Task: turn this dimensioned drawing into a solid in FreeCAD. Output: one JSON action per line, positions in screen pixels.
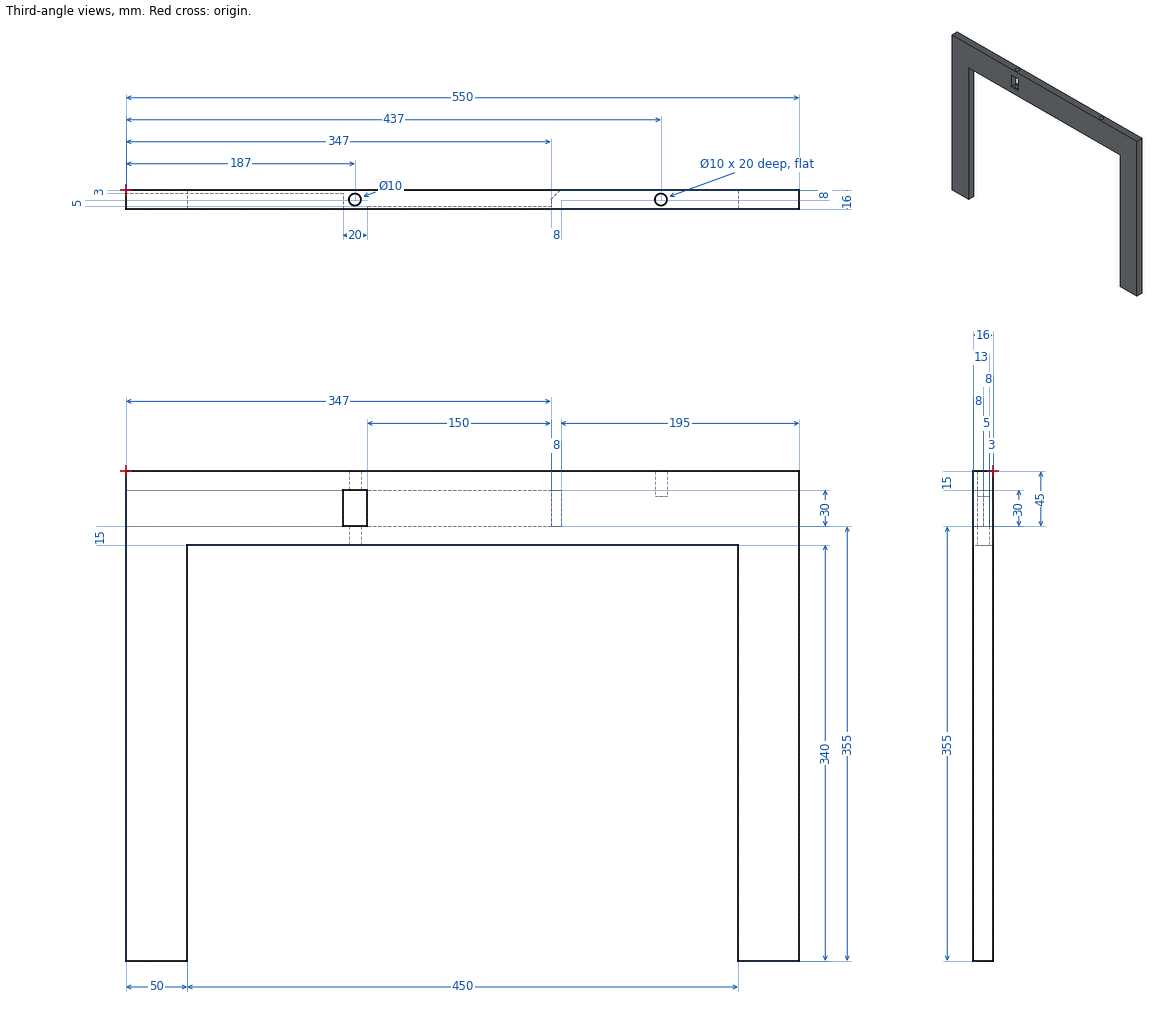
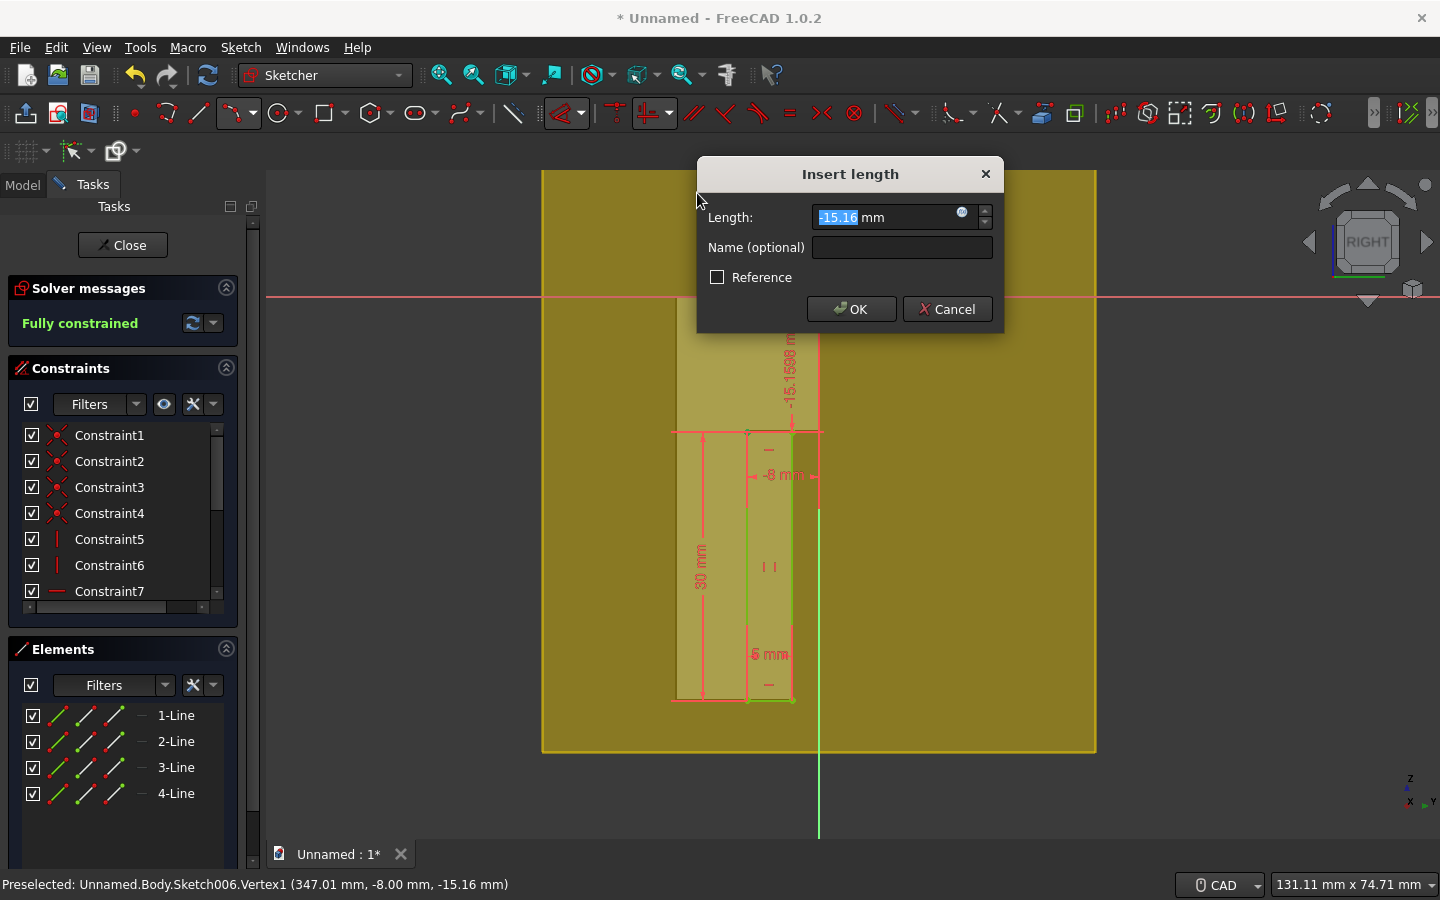
{"action": "type", "text": "-15"}
{"action": "key", "text": "Return"}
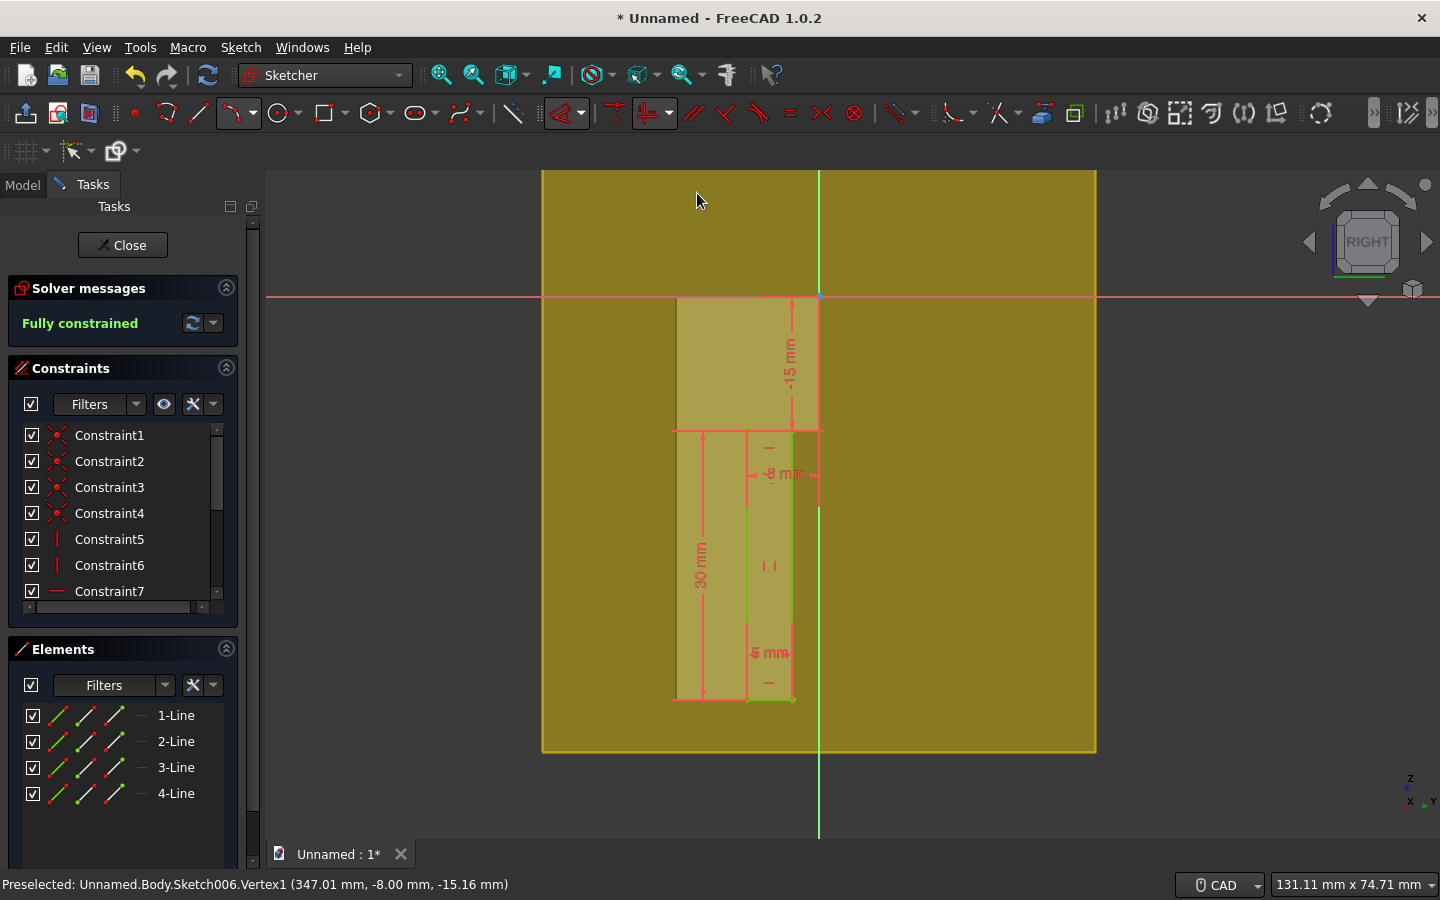
{"action": "left_click", "coordinate": [123, 245]}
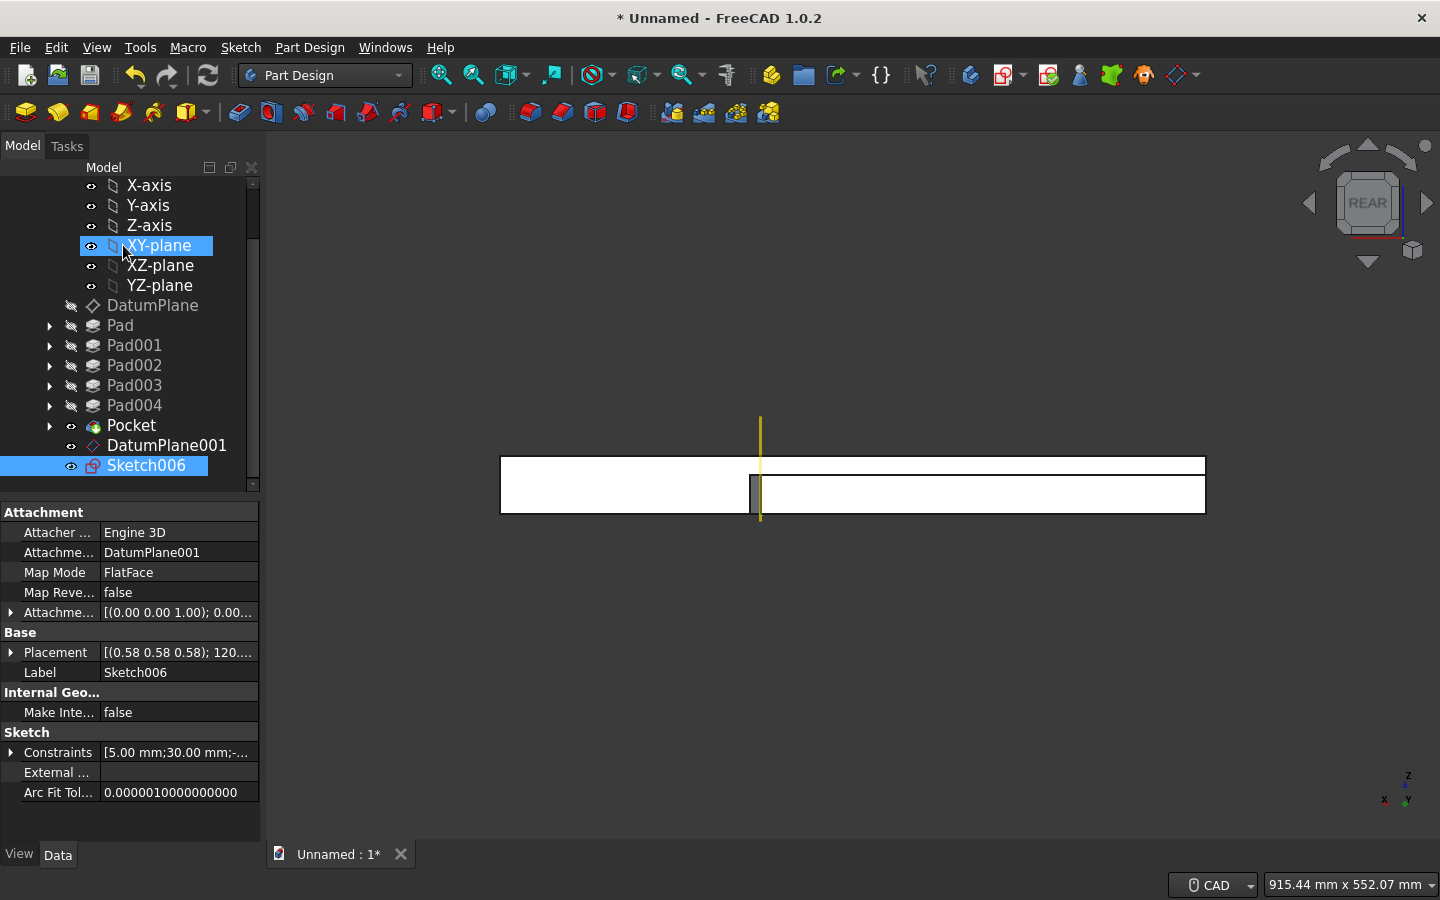
{"action": "left_click", "coordinate": [240, 112]}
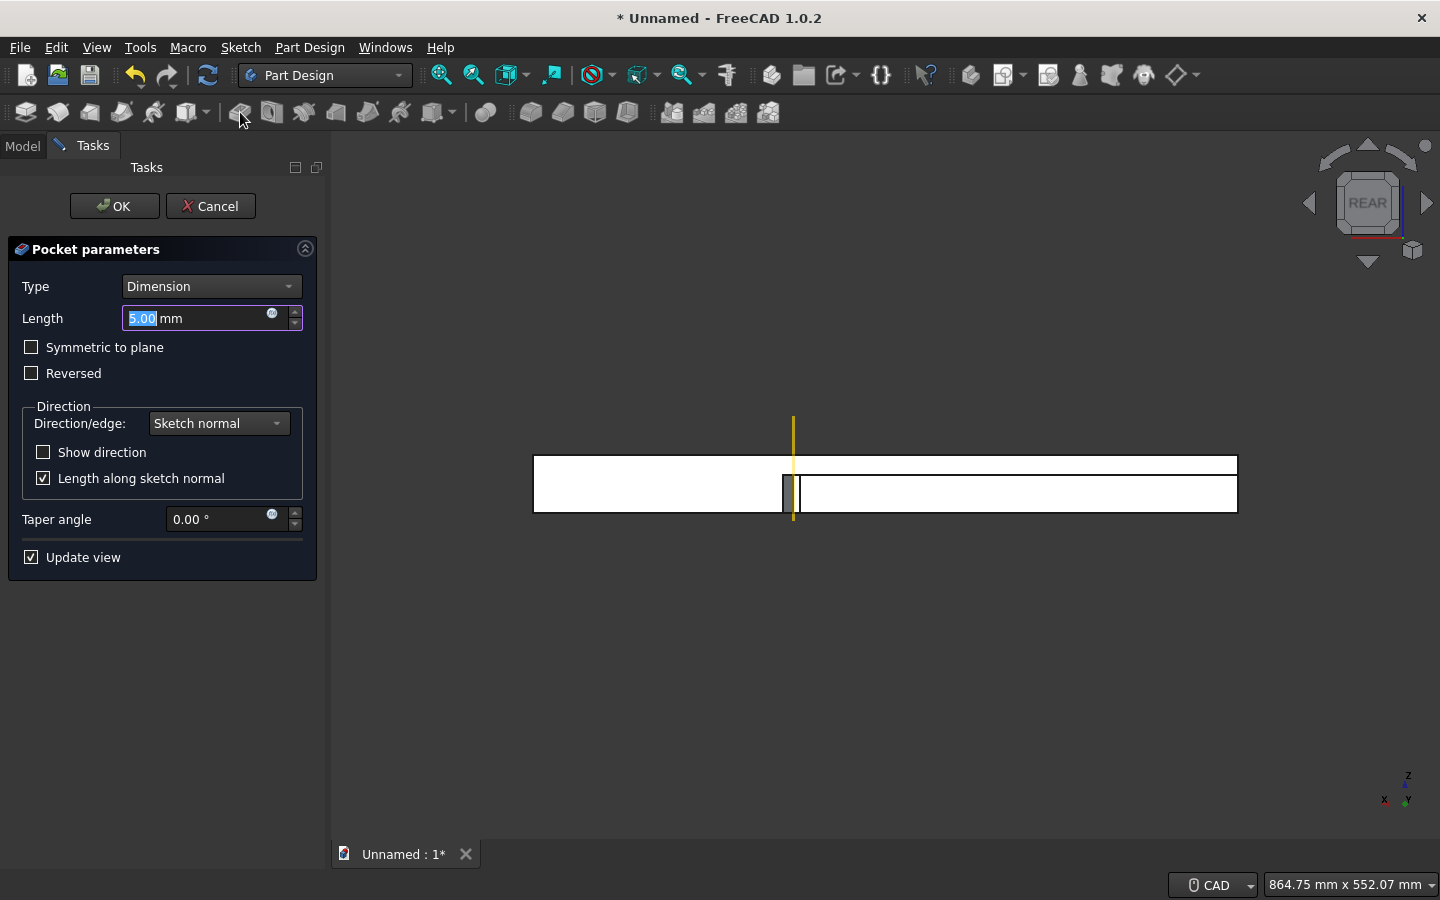
{"action": "type", "text": "150"}
{"action": "key", "text": "Tab"}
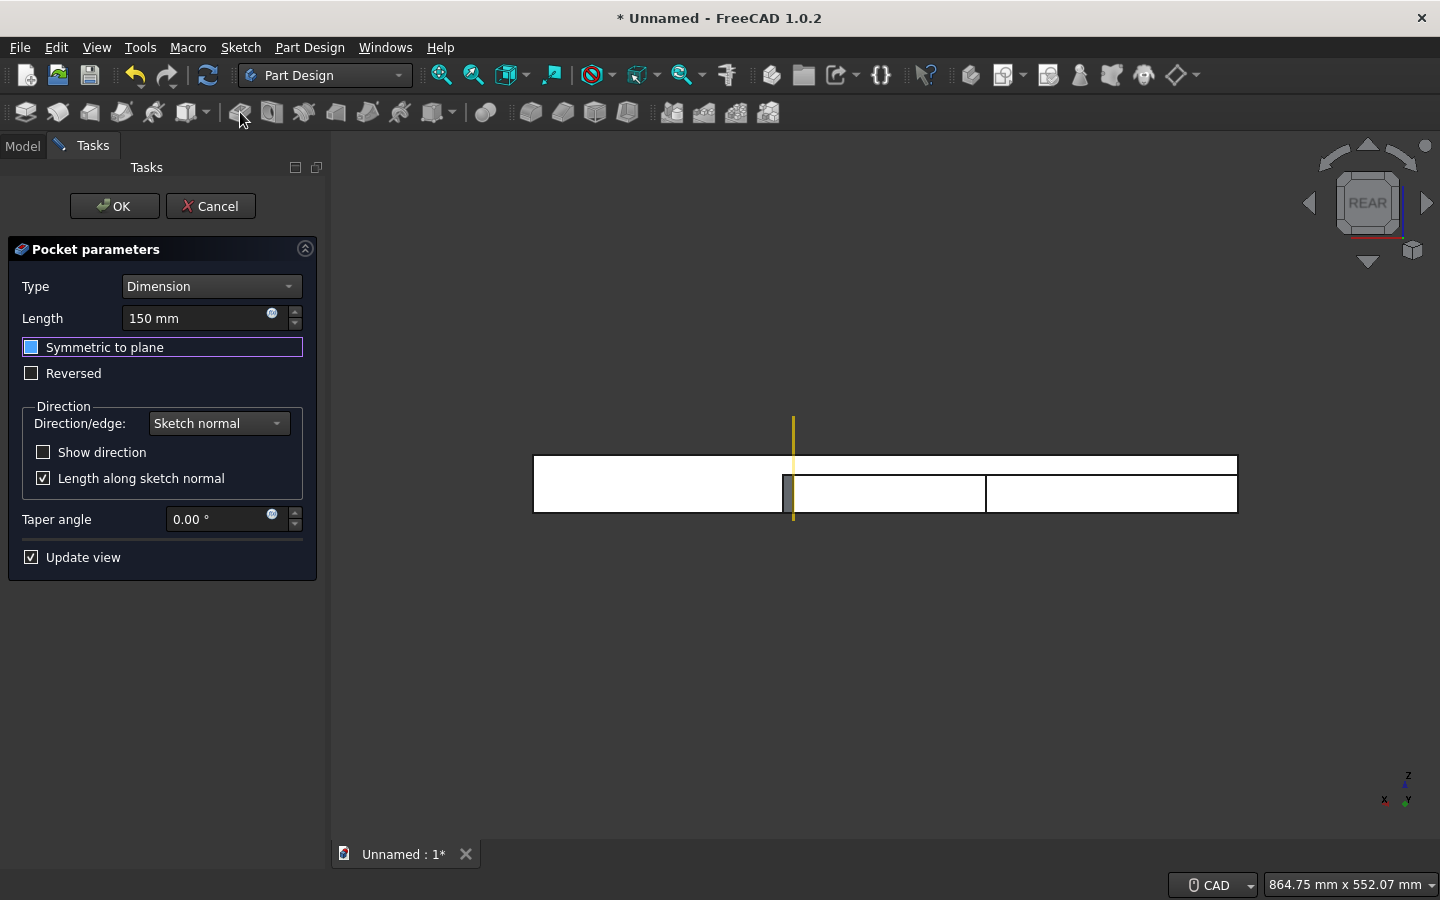
{"action": "left_click", "coordinate": [115, 206]}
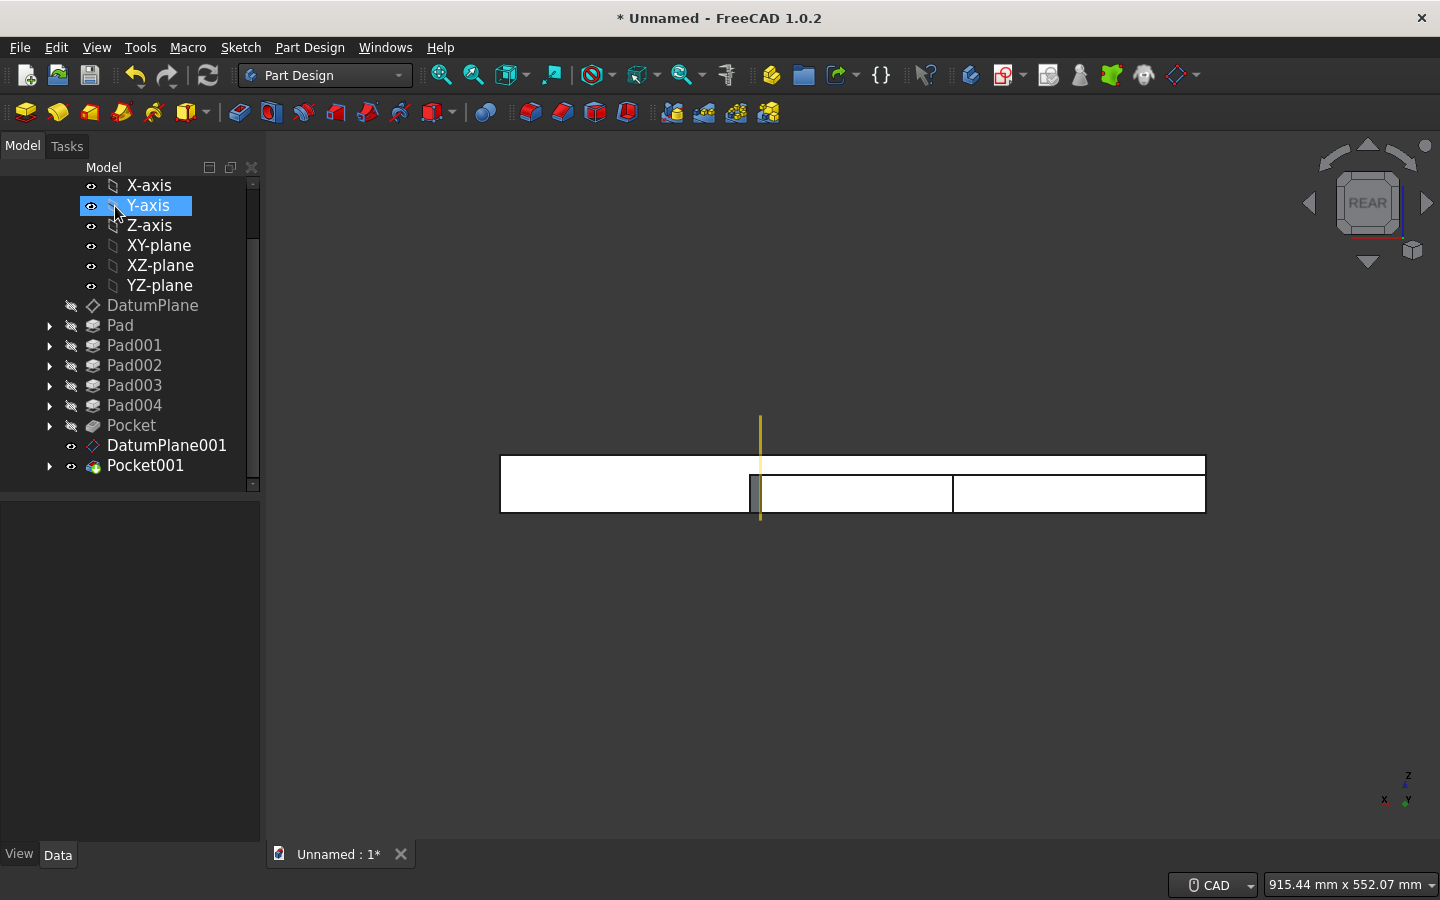
{"action": "left_click", "coordinate": [116, 446]}
{"action": "key", "text": "space"}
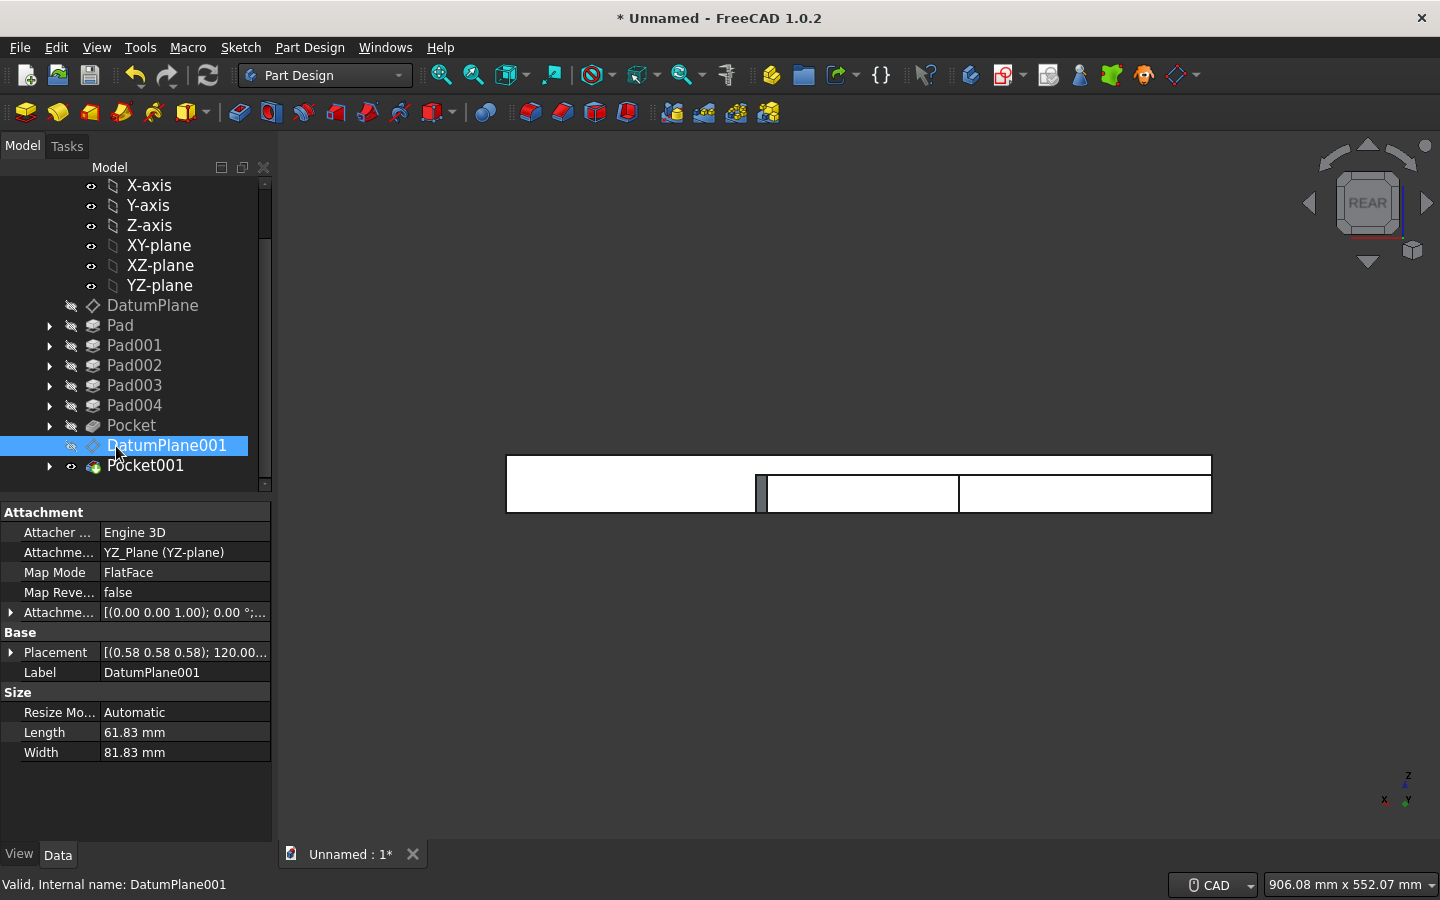
{"action": "scroll", "coordinate": [160, 321], "scroll_direction": "down", "scroll_amount": 3}